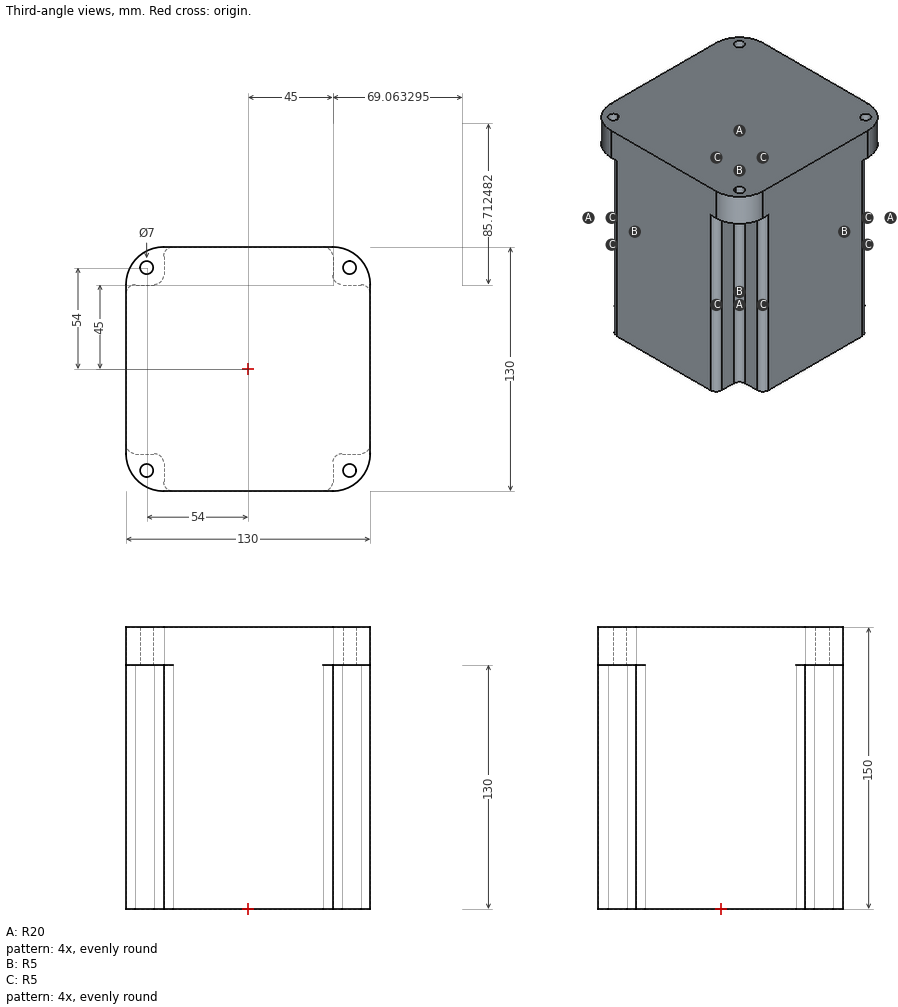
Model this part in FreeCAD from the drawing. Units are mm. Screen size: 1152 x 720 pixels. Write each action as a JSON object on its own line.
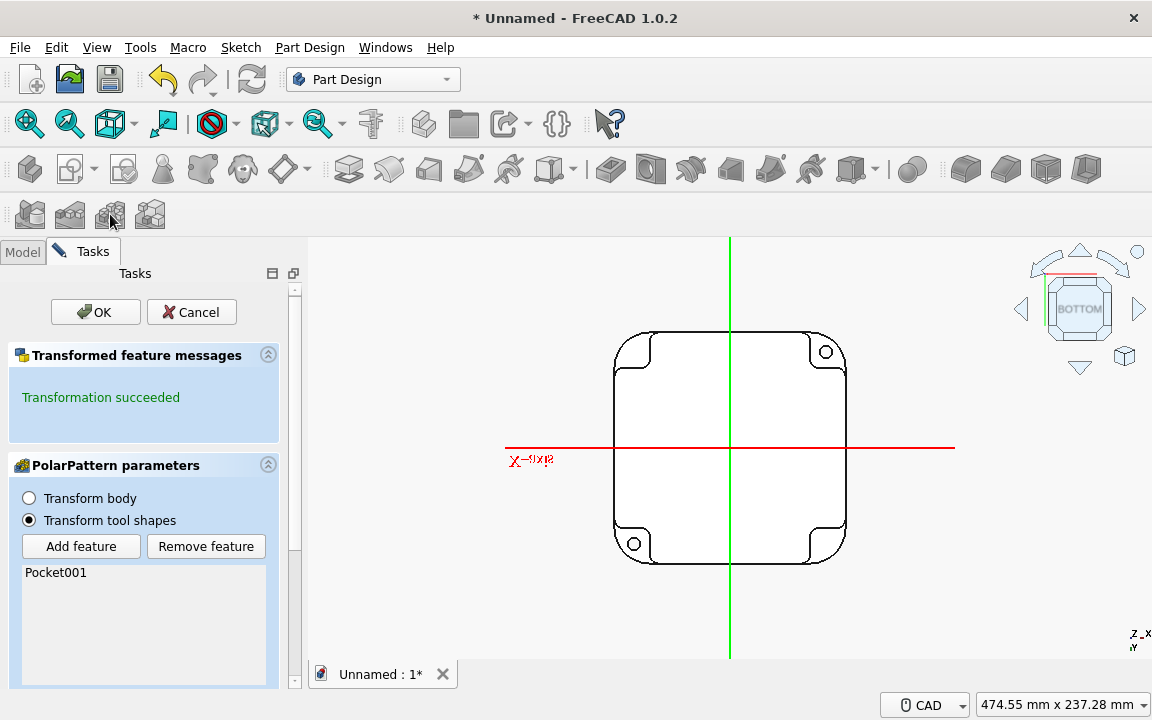
{"action": "scroll", "coordinate": [295, 486], "scroll_direction": "down", "scroll_amount": 2}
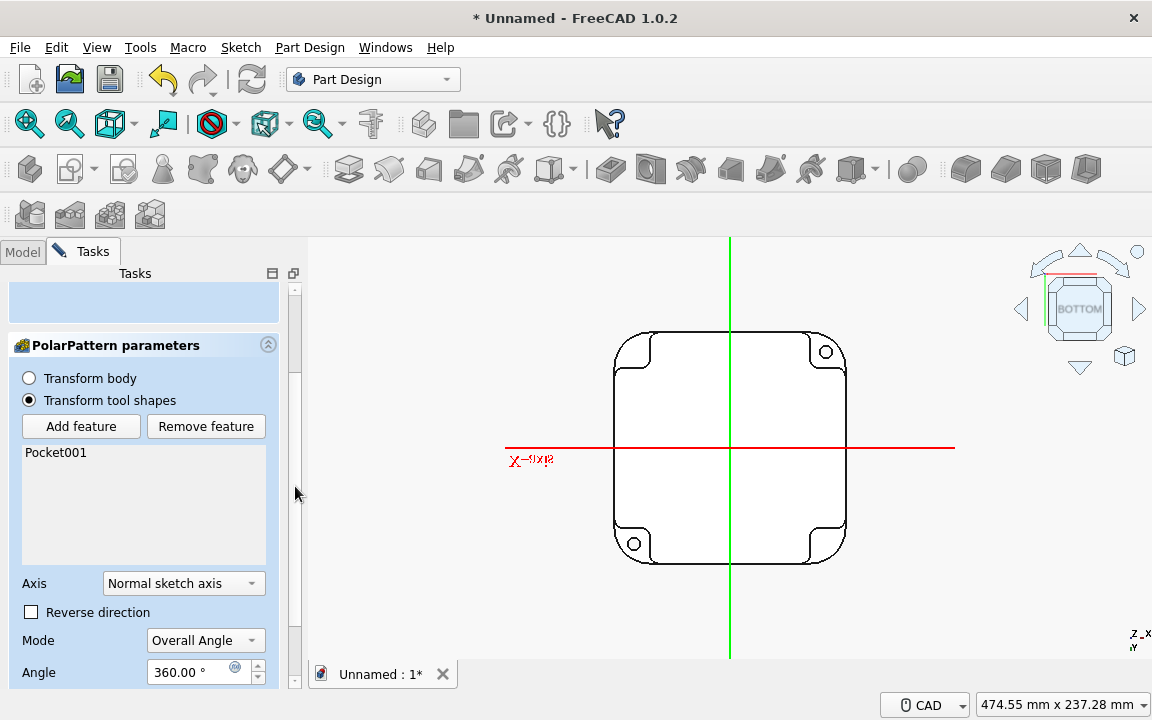
{"action": "left_click", "coordinate": [184, 584]}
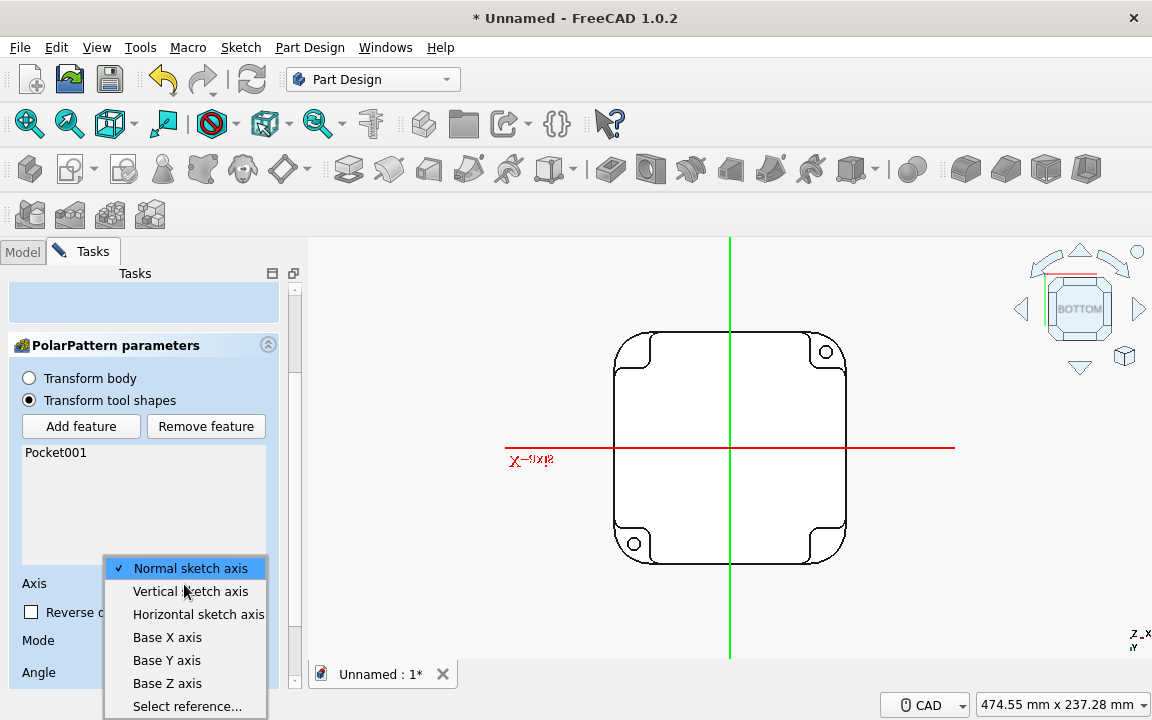
{"action": "left_click", "coordinate": [184, 684]}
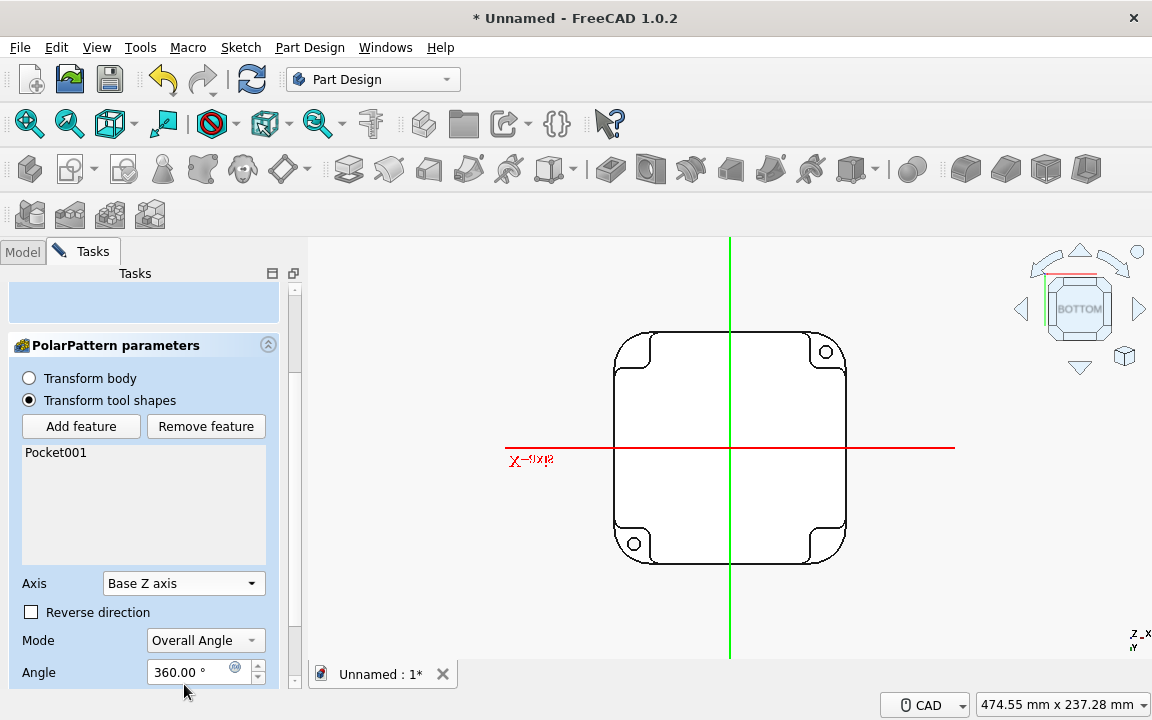
{"action": "scroll", "coordinate": [295, 486], "scroll_direction": "down", "scroll_amount": 2}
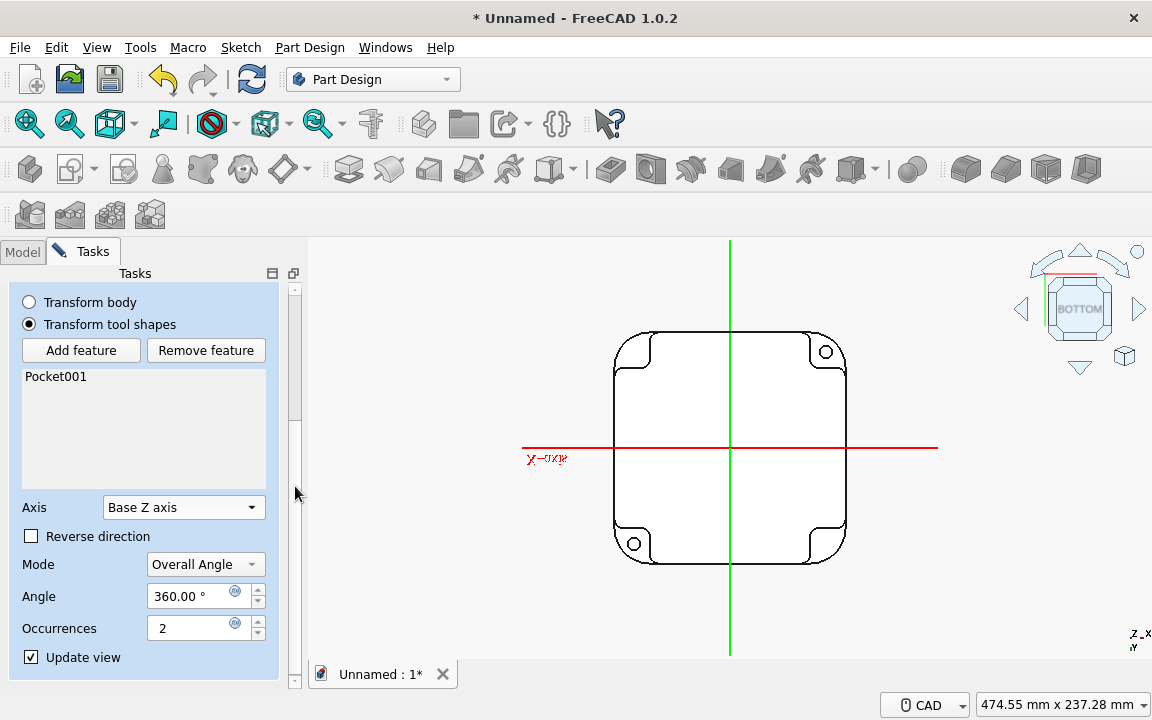
{"action": "triple_click", "coordinate": [198, 628]}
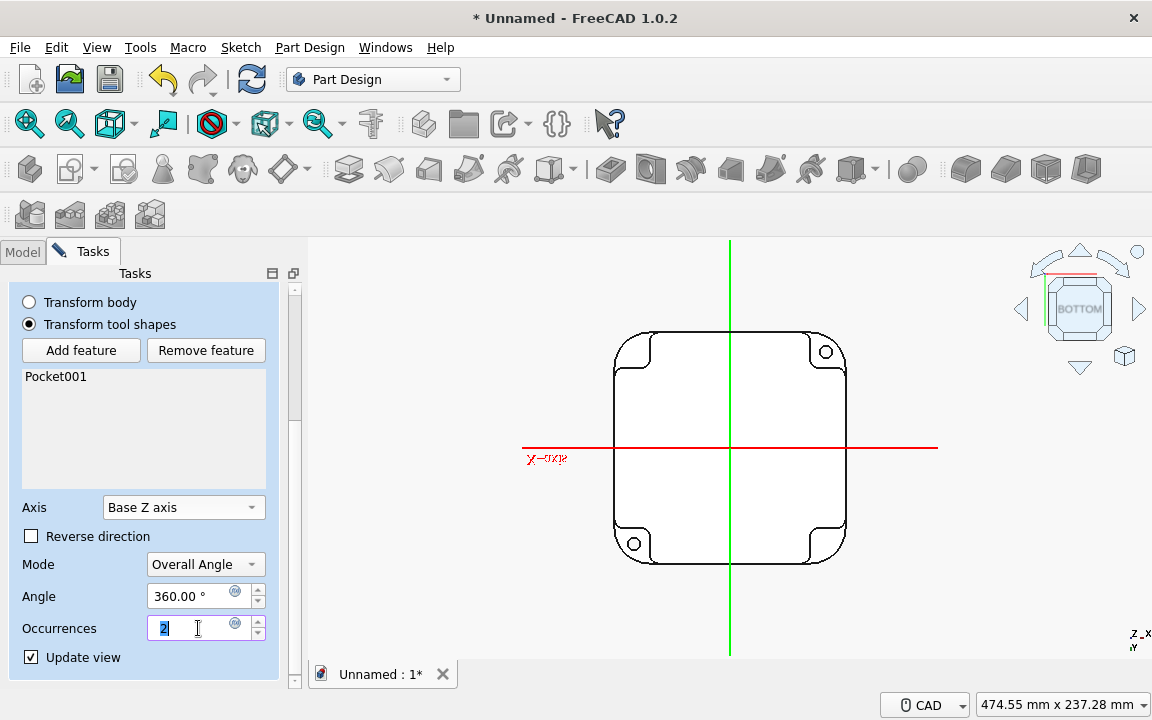
{"action": "type", "text": "4"}
{"action": "key", "text": "Tab"}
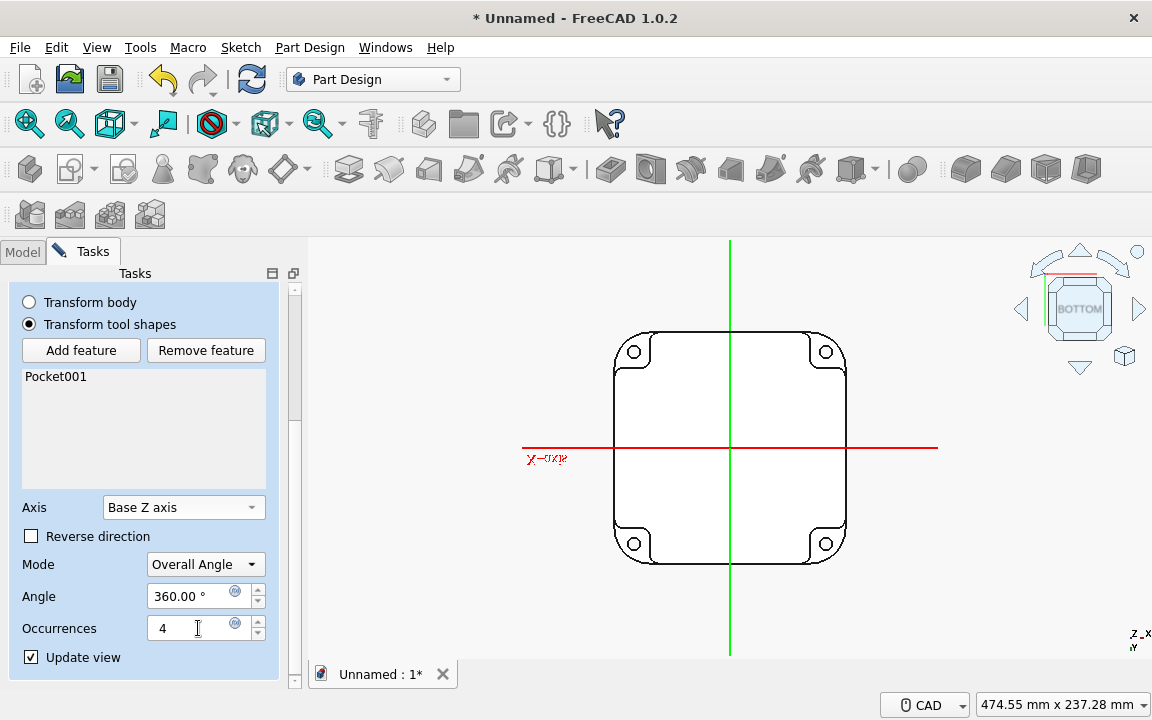
{"action": "scroll", "coordinate": [295, 486], "scroll_direction": "up", "scroll_amount": 5}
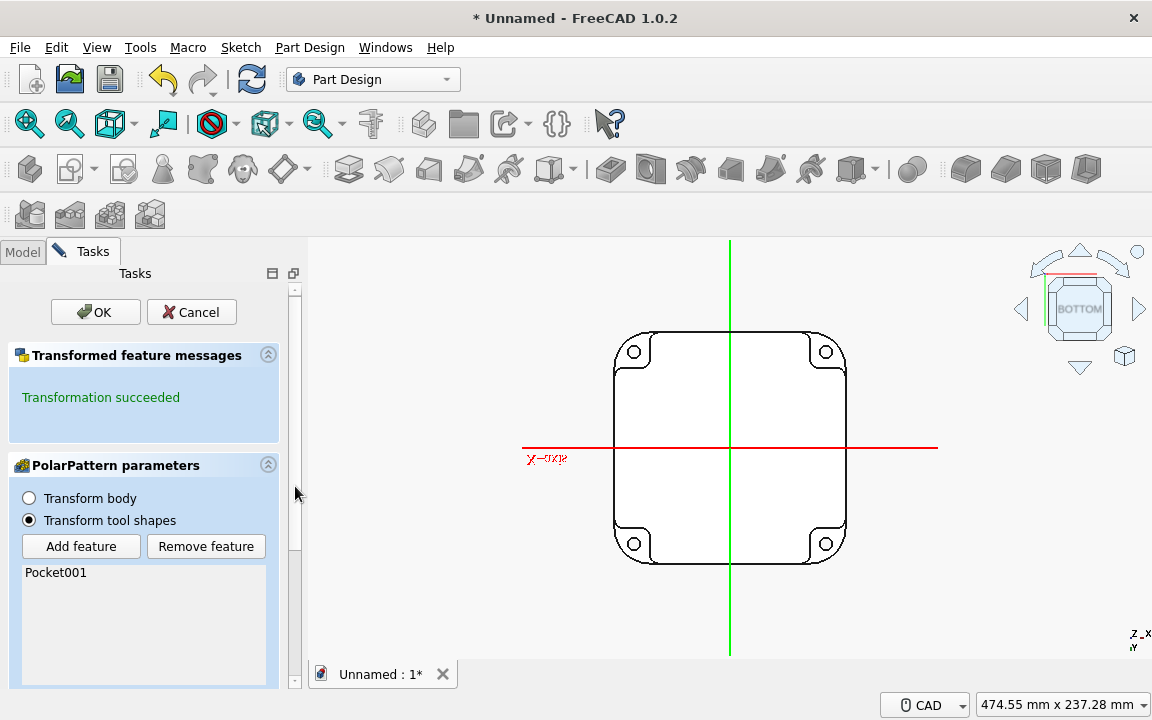
{"action": "left_click", "coordinate": [96, 312]}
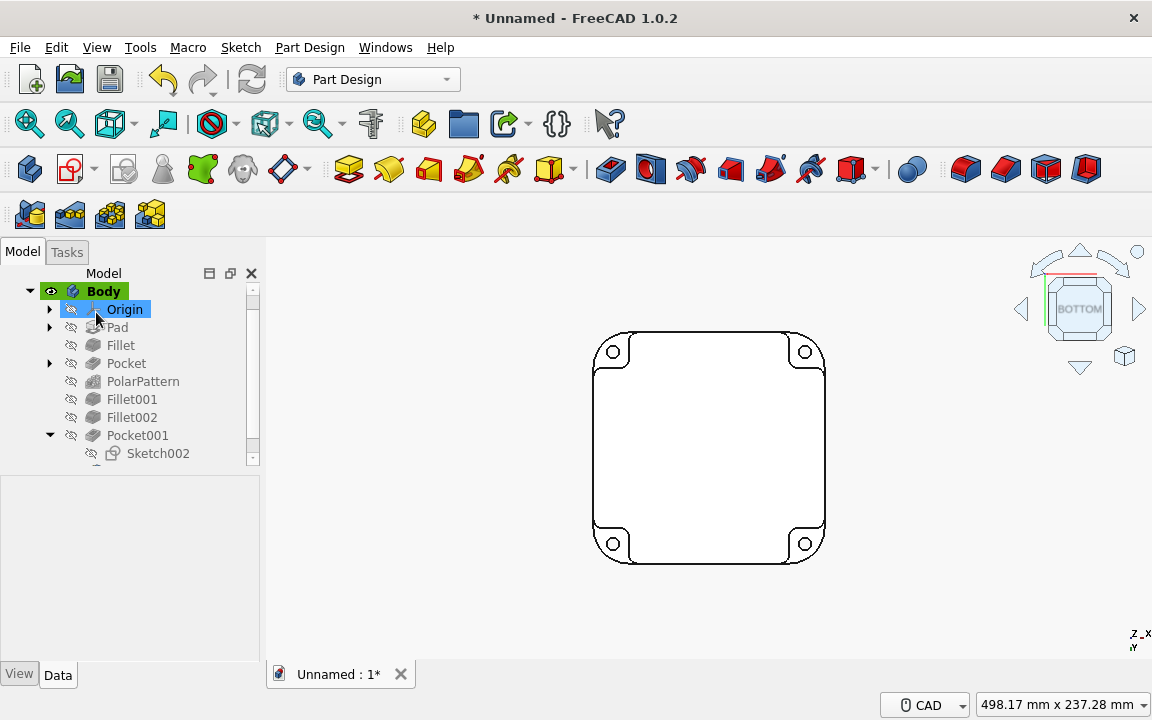
{"action": "key", "text": "0"}